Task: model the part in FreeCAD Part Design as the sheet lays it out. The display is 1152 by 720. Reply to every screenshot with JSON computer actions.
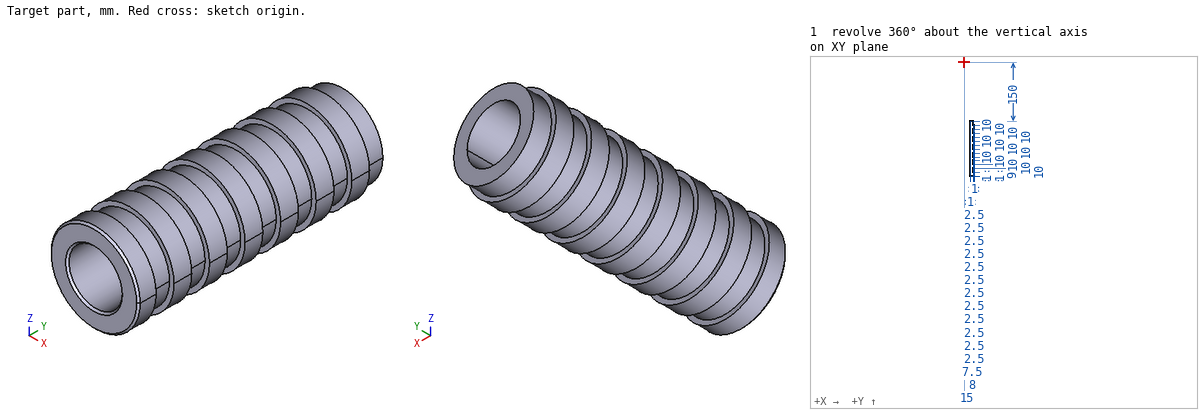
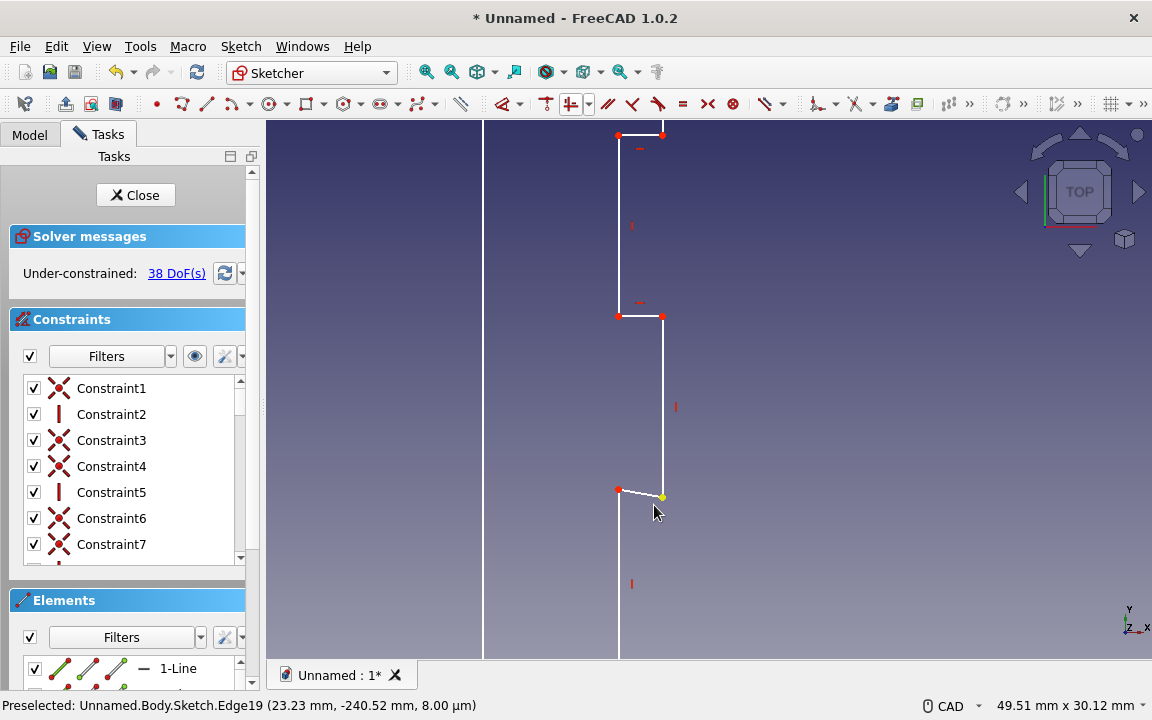
{"action": "left_click", "coordinate": [649, 495]}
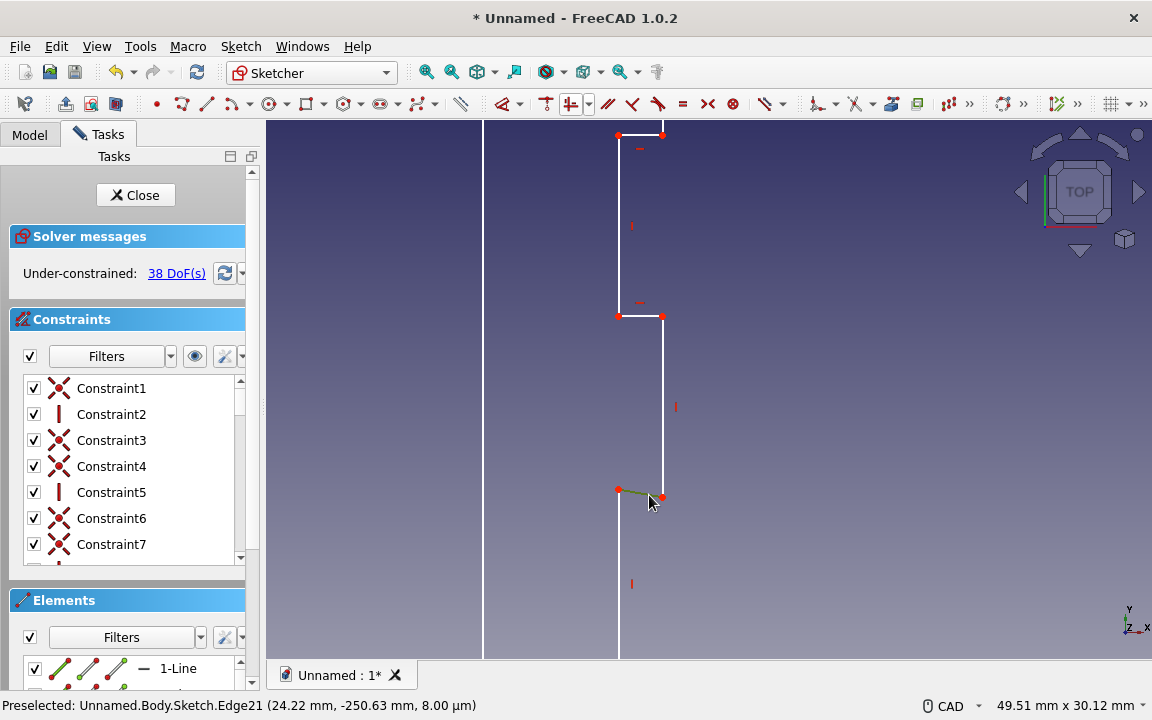
{"action": "key", "text": "h"}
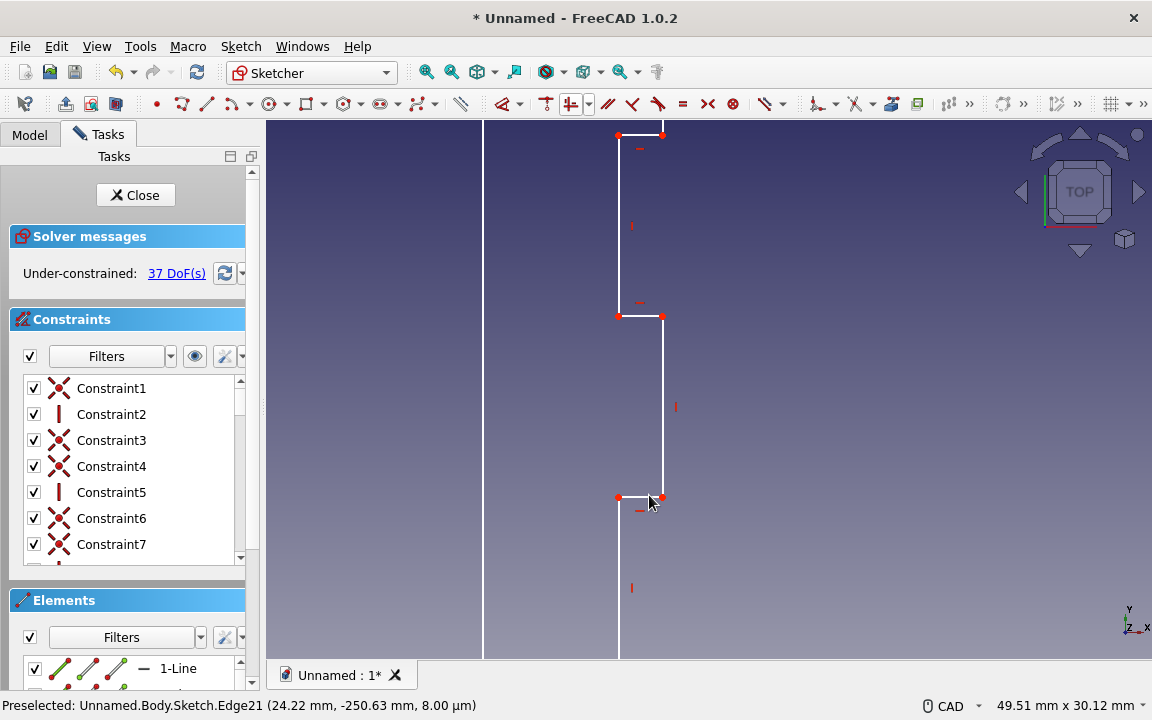
{"action": "scroll", "coordinate": [654, 505], "scroll_direction": "down", "scroll_amount": 14}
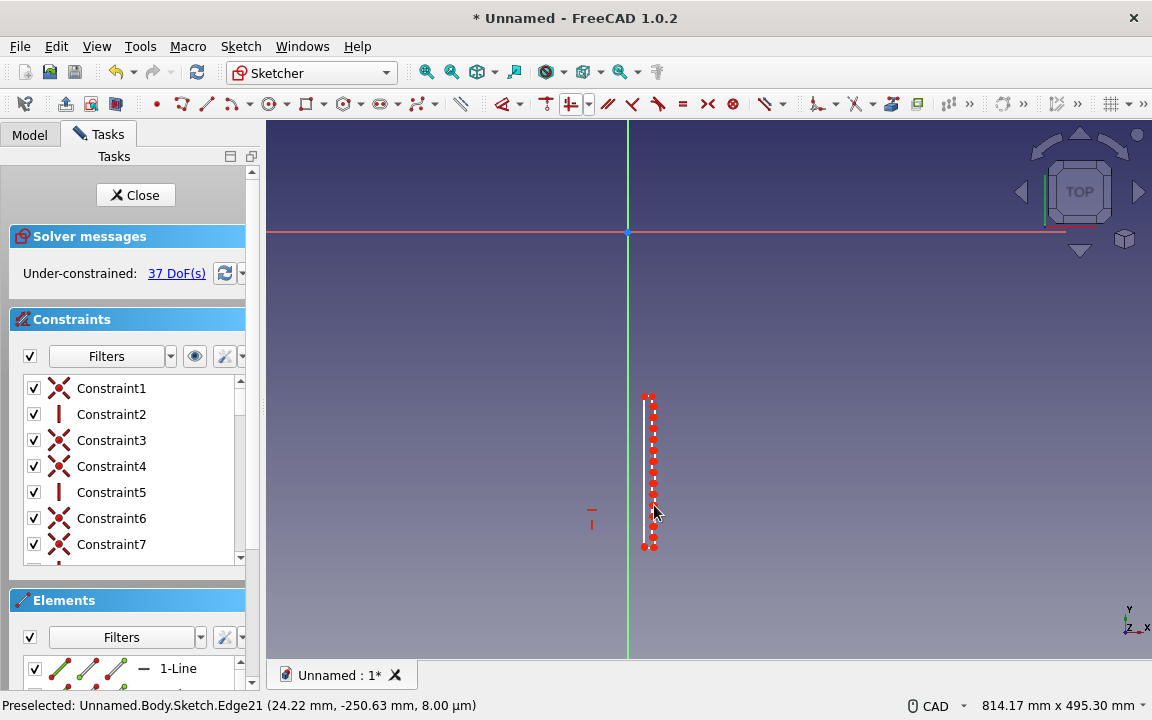
{"action": "scroll", "coordinate": [653, 516], "scroll_direction": "up", "scroll_amount": 14}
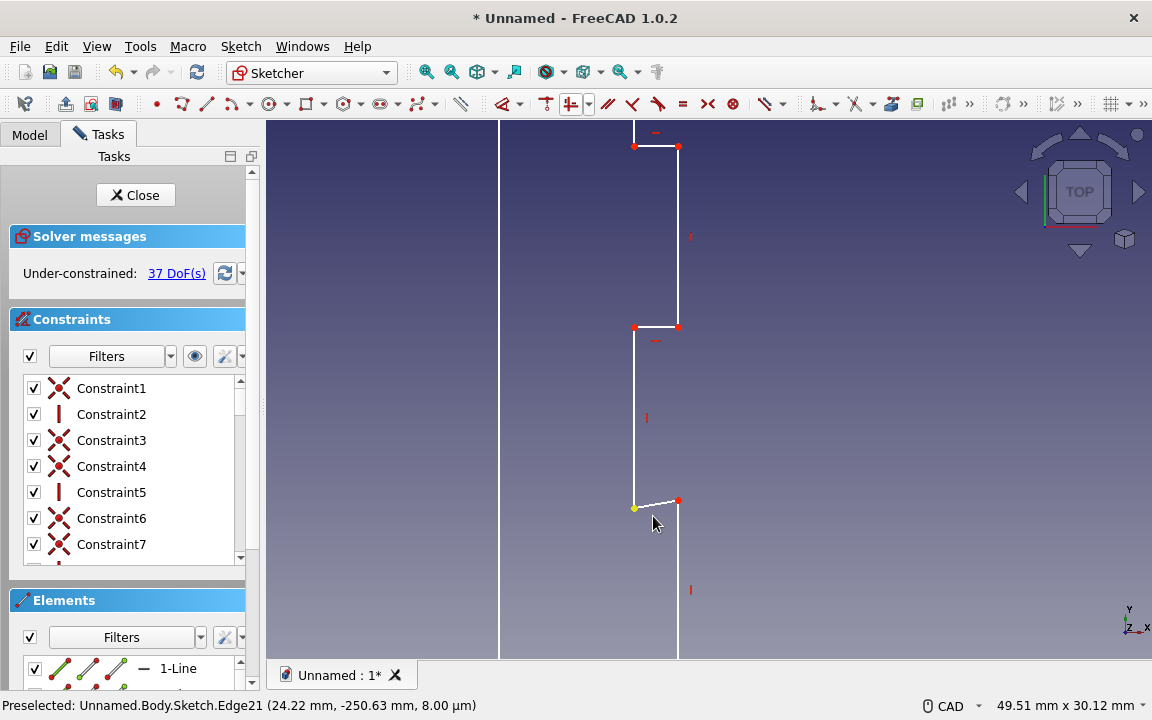
{"action": "left_click", "coordinate": [647, 506]}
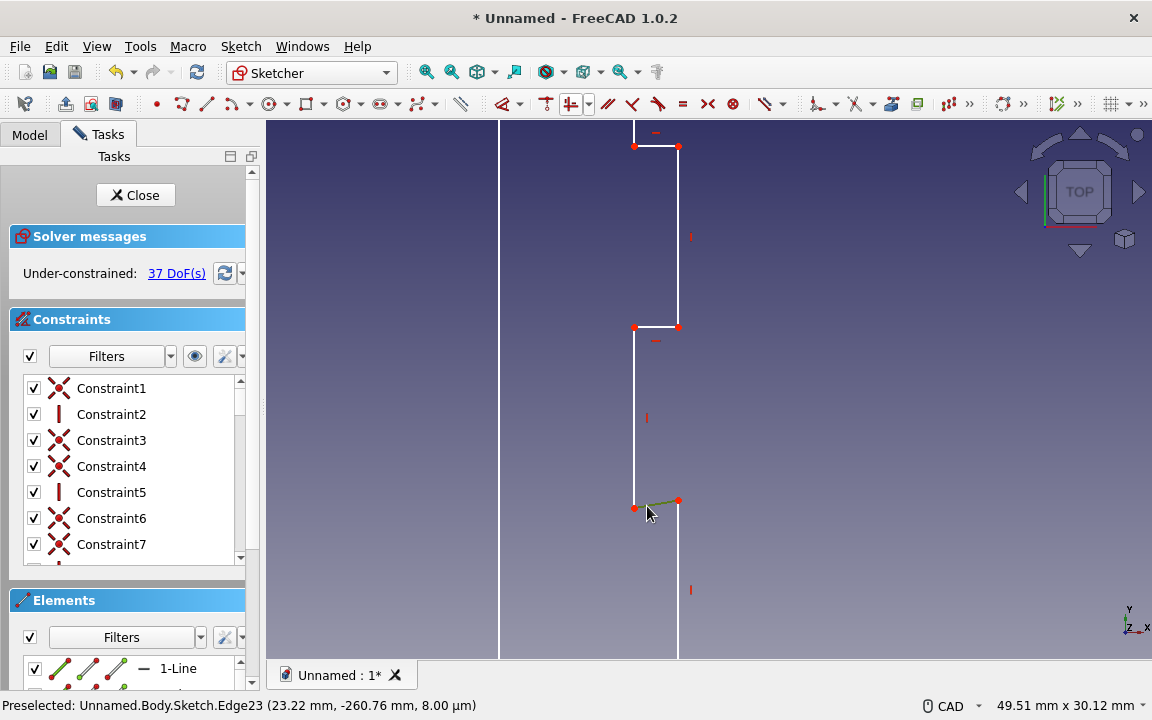
{"action": "key", "text": "h"}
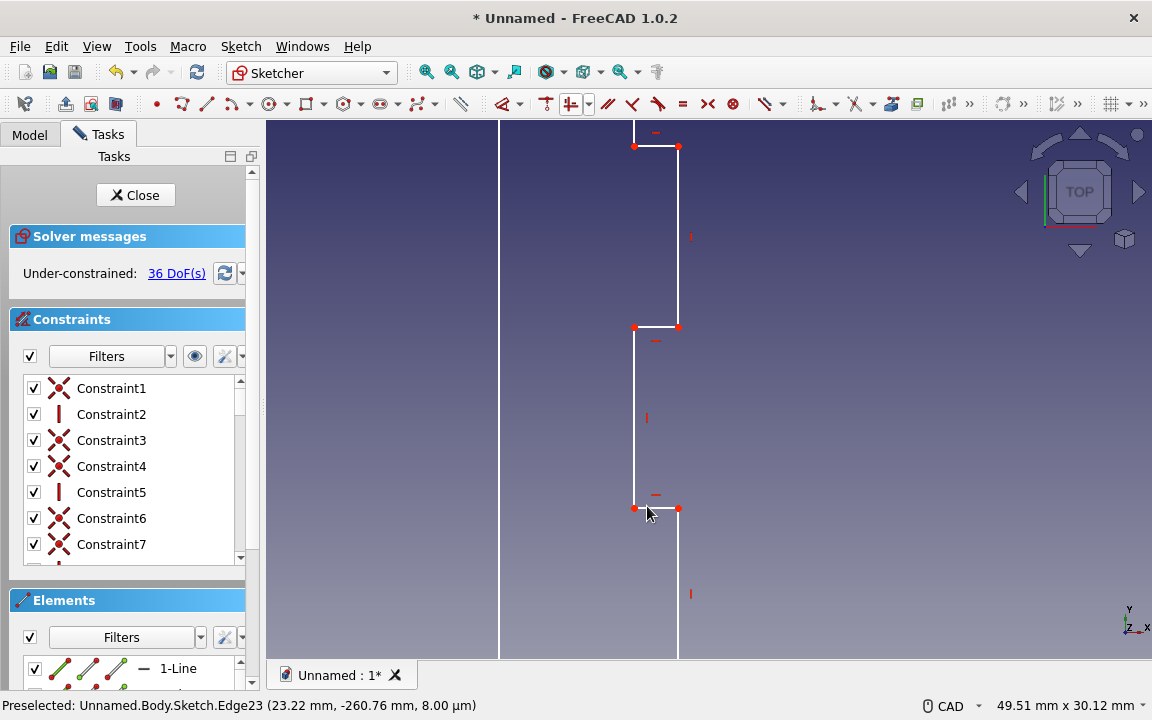
{"action": "scroll", "coordinate": [653, 516], "scroll_direction": "down", "scroll_amount": 14}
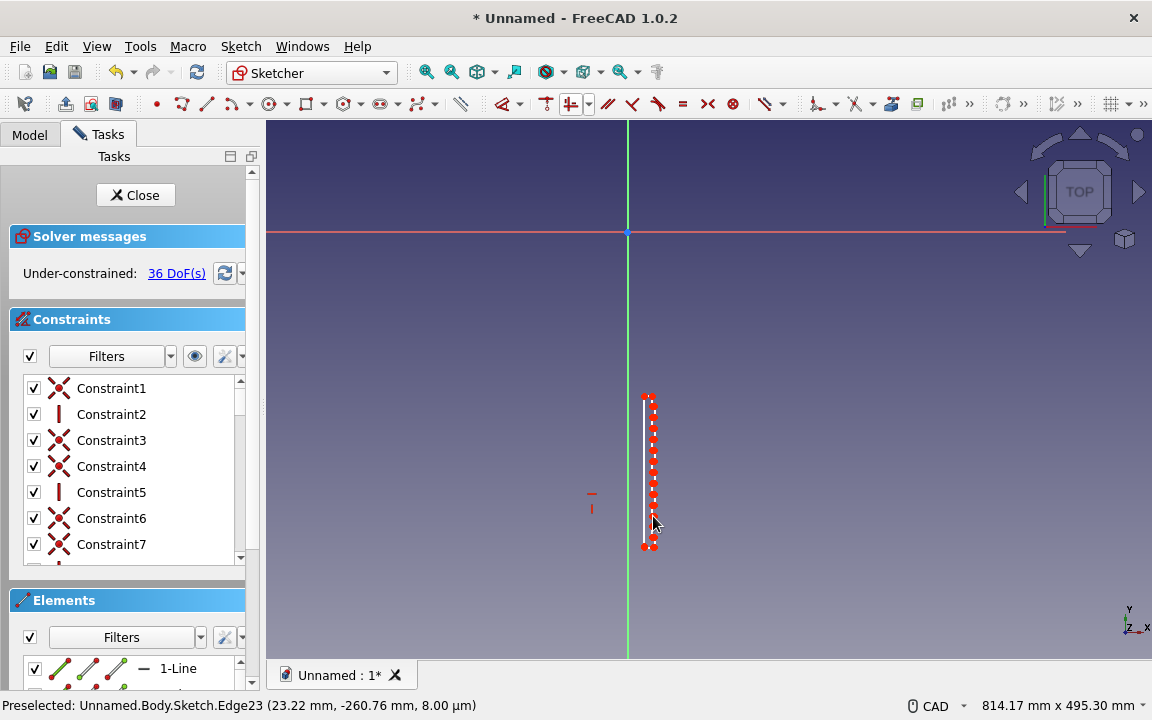
{"action": "scroll", "coordinate": [654, 526], "scroll_direction": "up", "scroll_amount": 14}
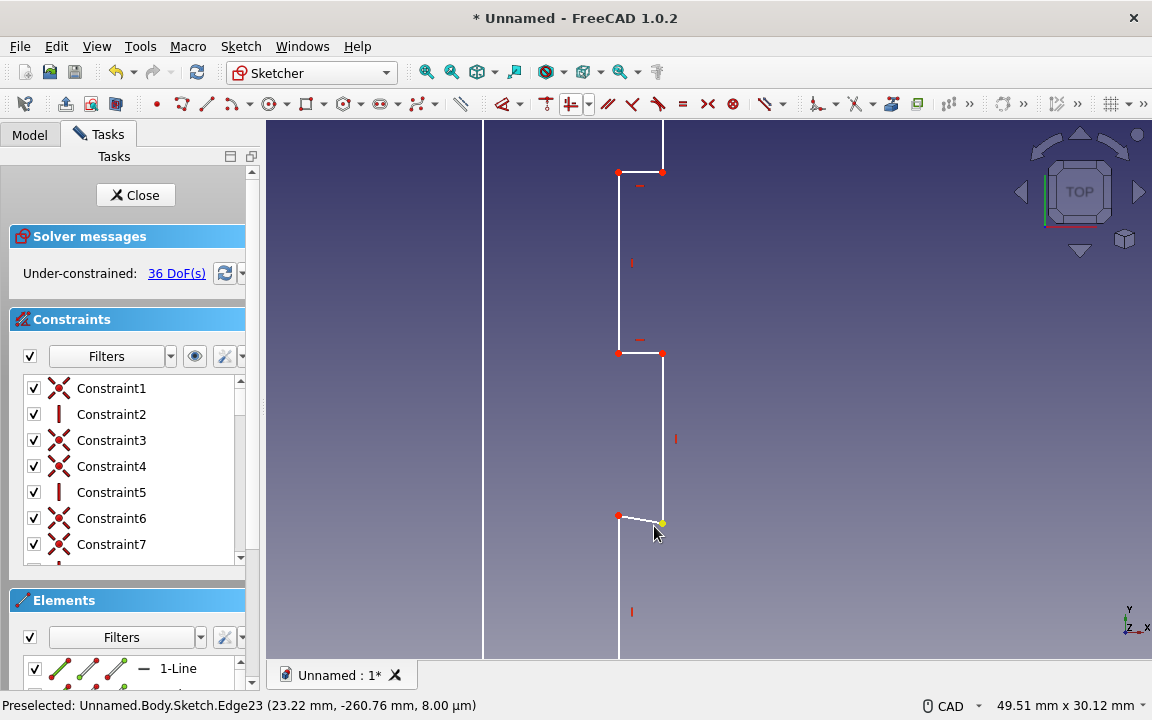
{"action": "left_click", "coordinate": [649, 521]}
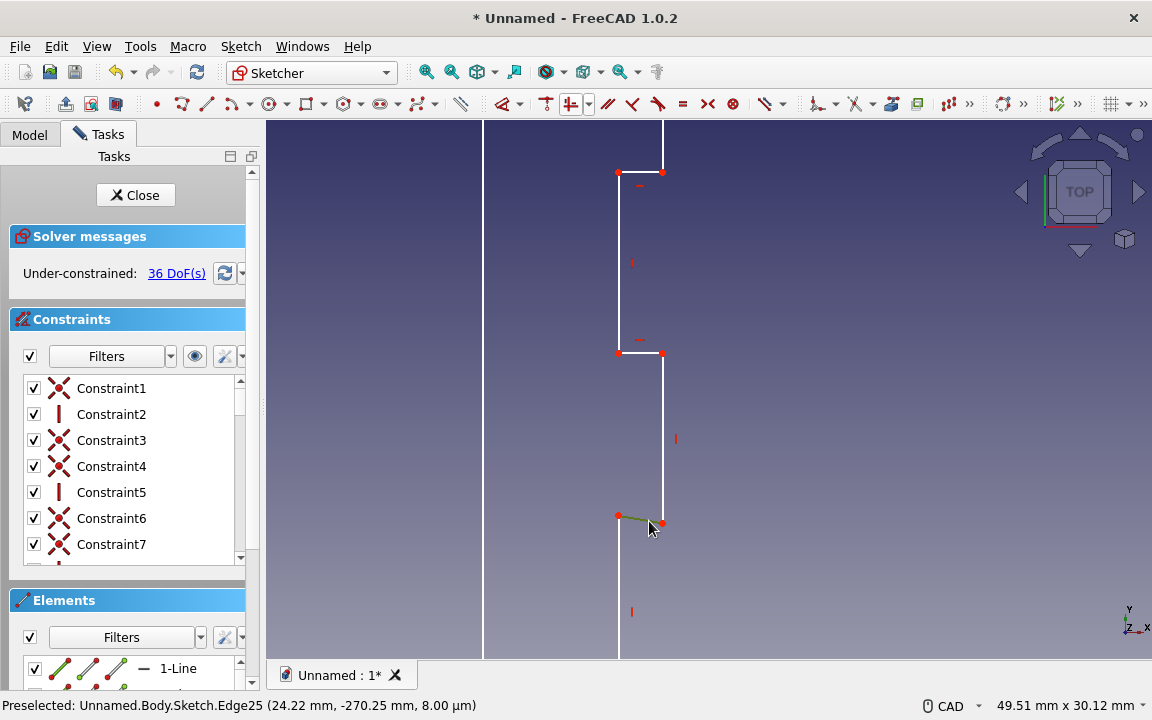
{"action": "key", "text": "h"}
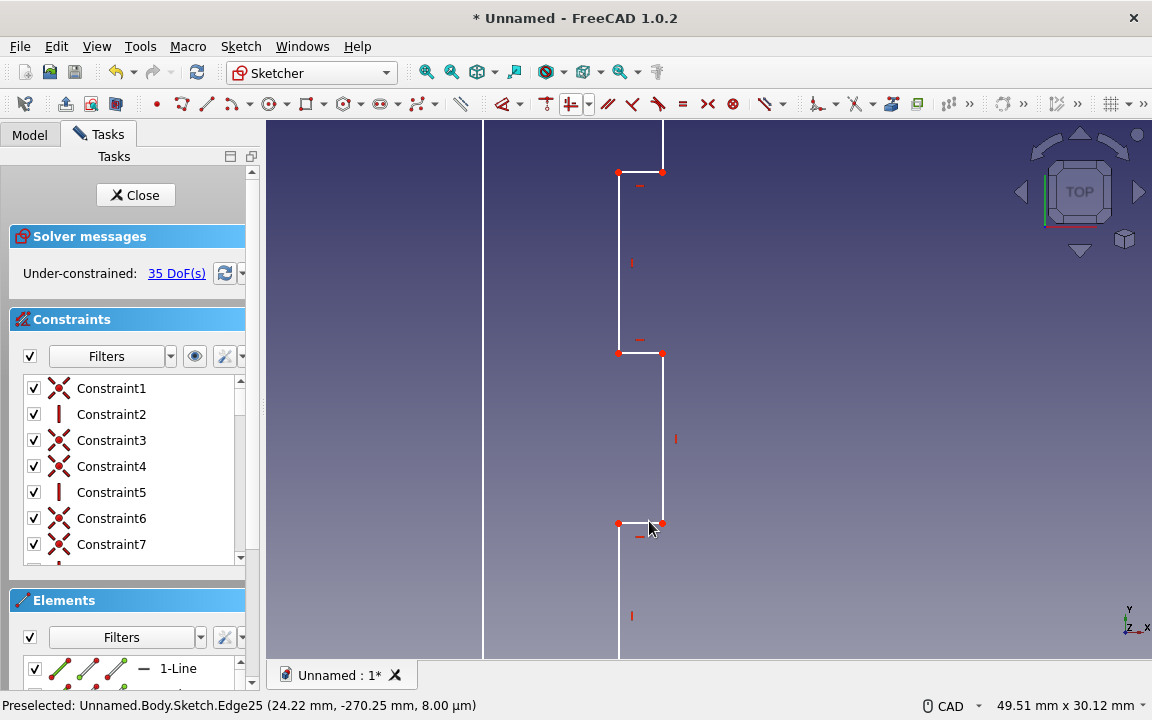
{"action": "scroll", "coordinate": [654, 526], "scroll_direction": "down", "scroll_amount": 14}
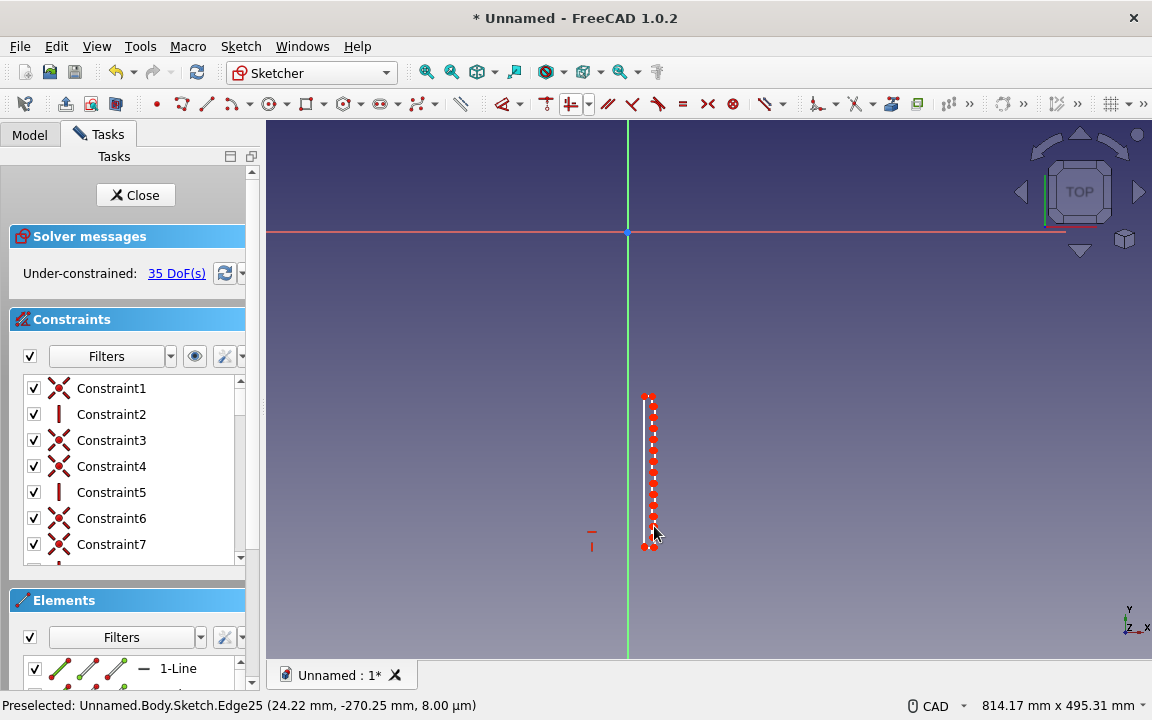
{"action": "scroll", "coordinate": [653, 538], "scroll_direction": "up", "scroll_amount": 14}